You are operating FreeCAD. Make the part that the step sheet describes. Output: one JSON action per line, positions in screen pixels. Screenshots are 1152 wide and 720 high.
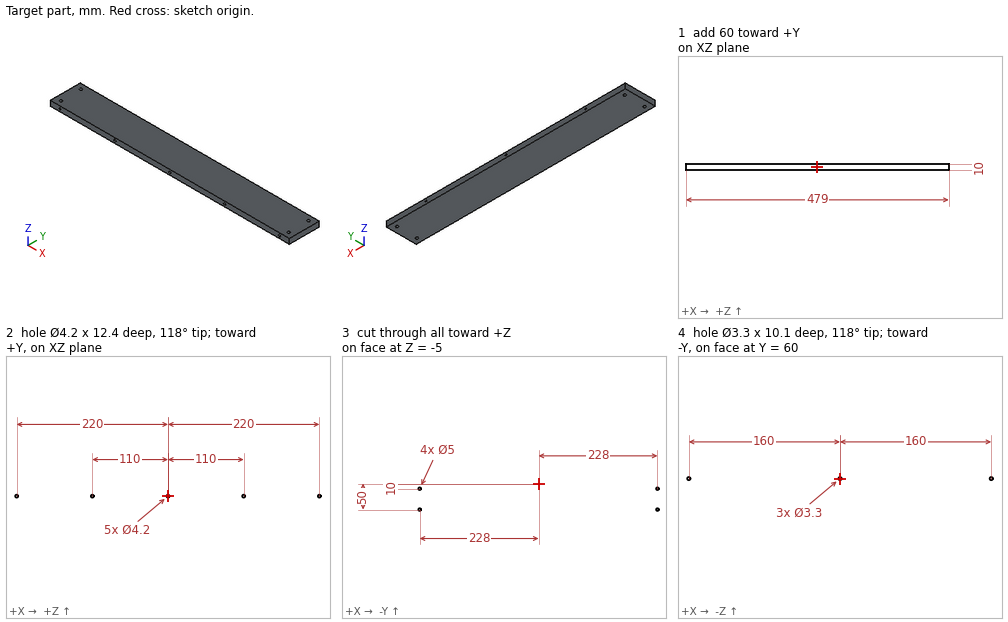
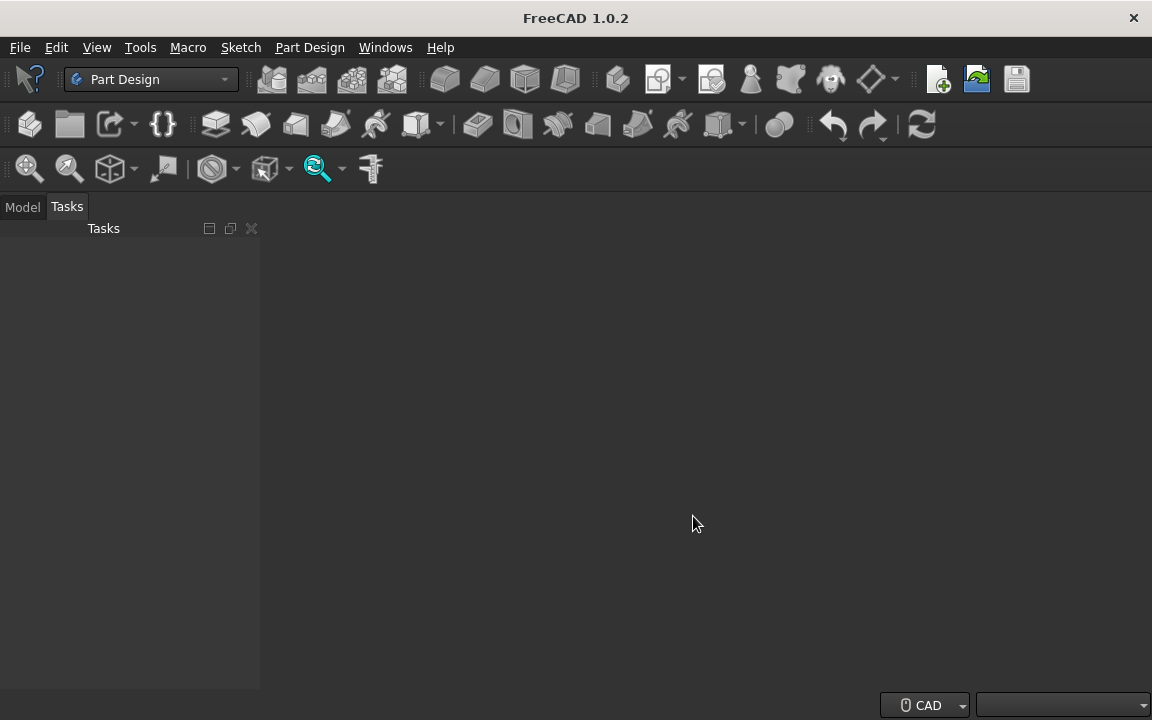
{"action": "left_click", "coordinate": [938, 80]}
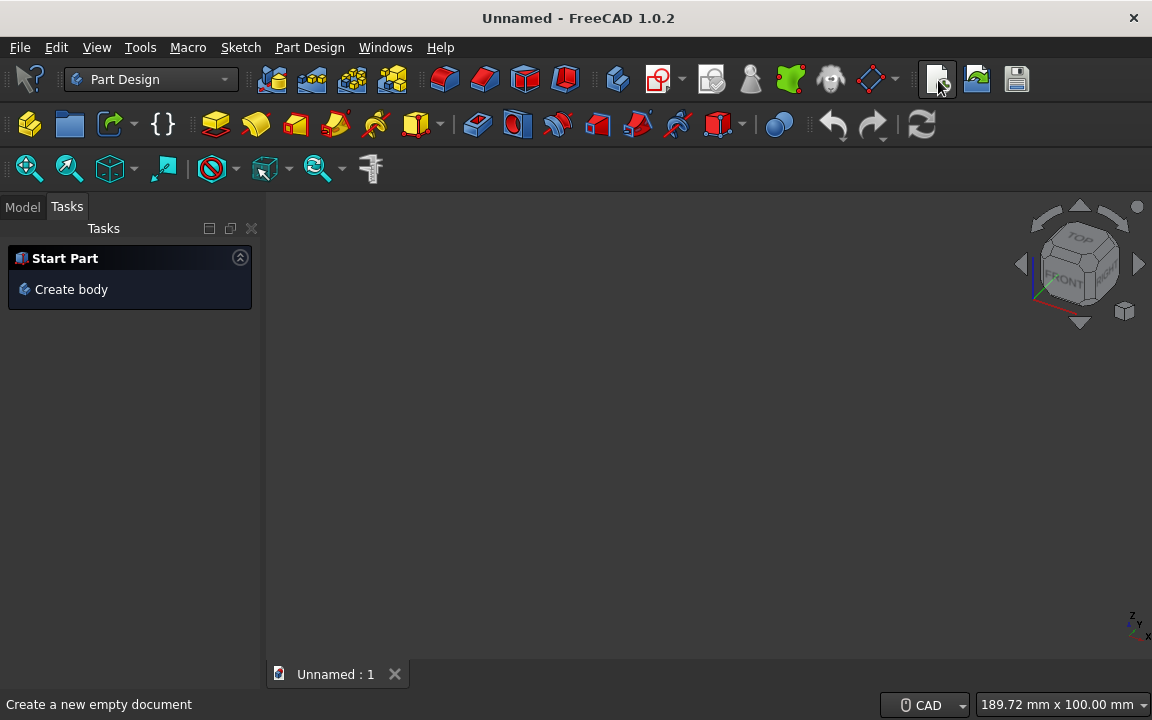
{"action": "left_click", "coordinate": [658, 80]}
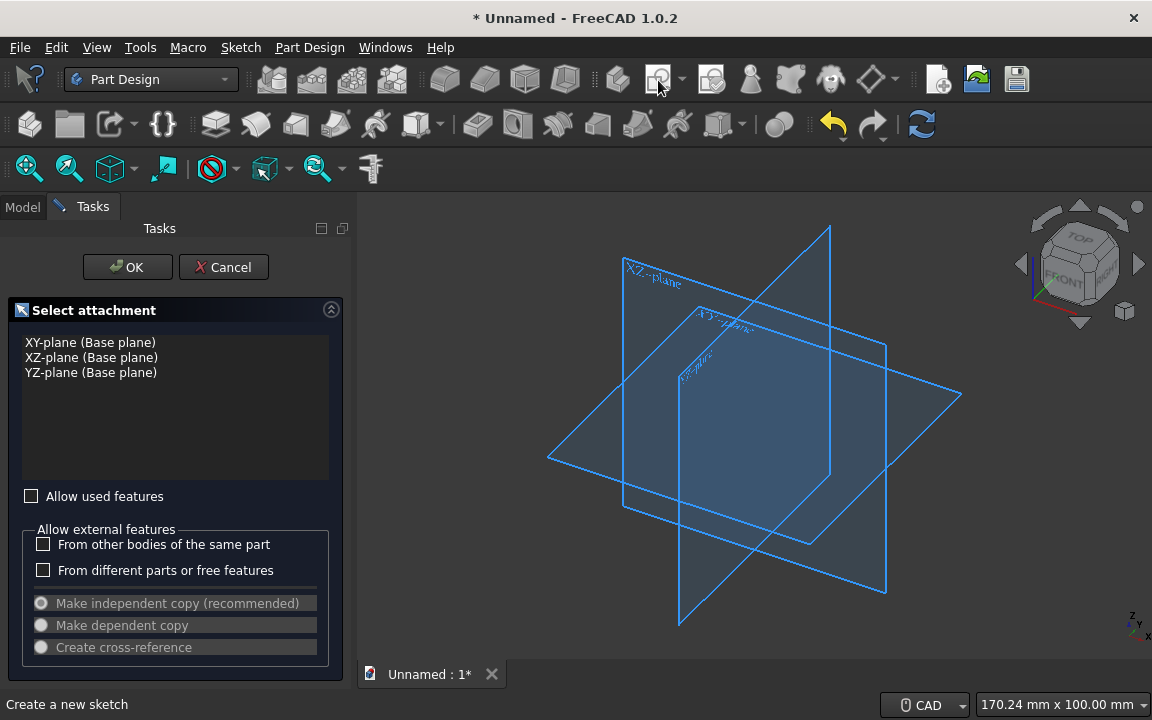
{"action": "left_click", "coordinate": [82, 358]}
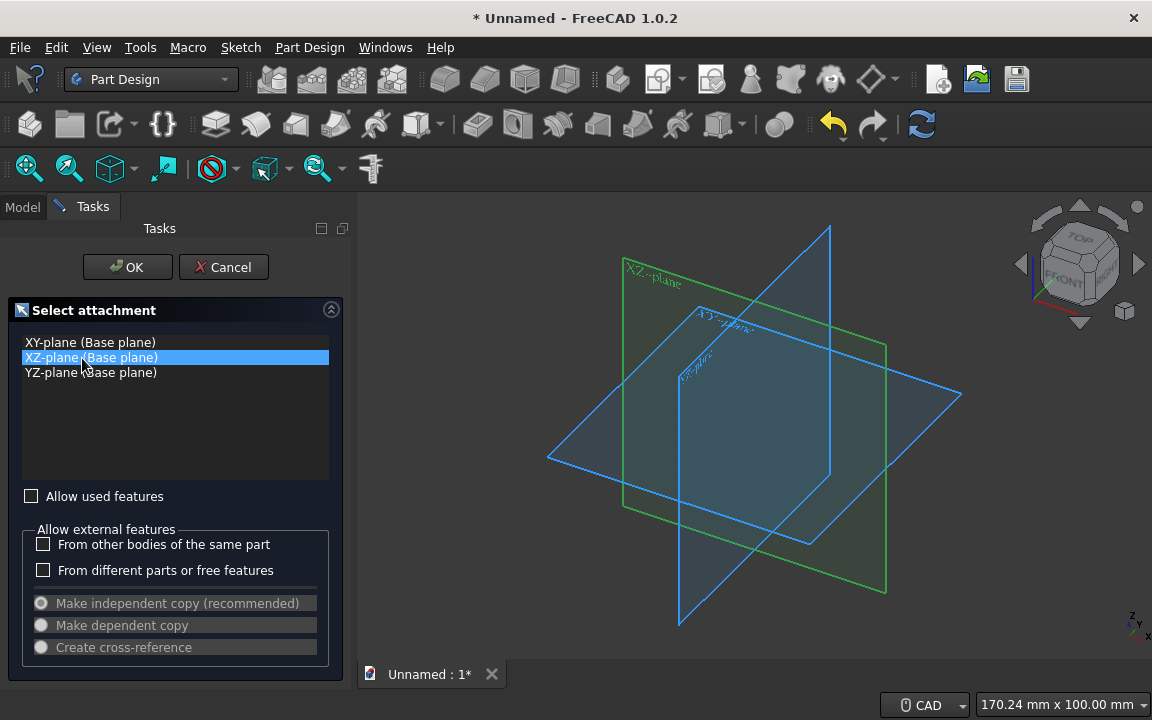
{"action": "left_click", "coordinate": [128, 267]}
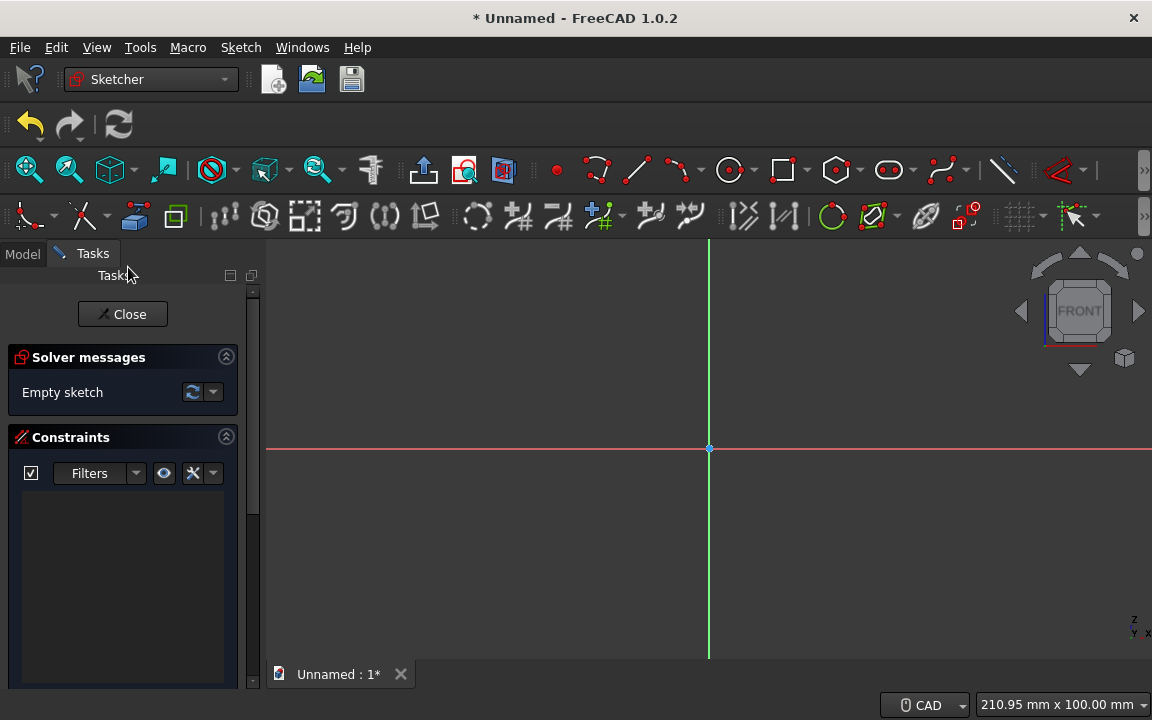
{"action": "scroll", "coordinate": [618, 449], "scroll_direction": "down", "scroll_amount": 7}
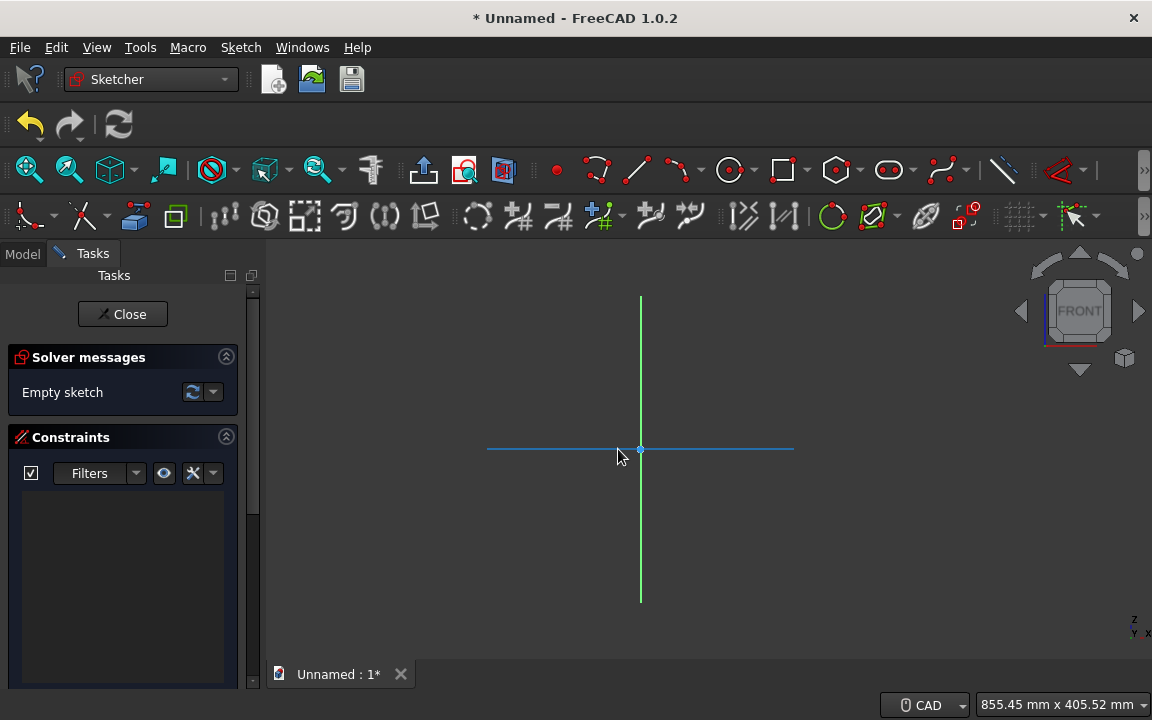
{"action": "left_click", "coordinate": [810, 170]}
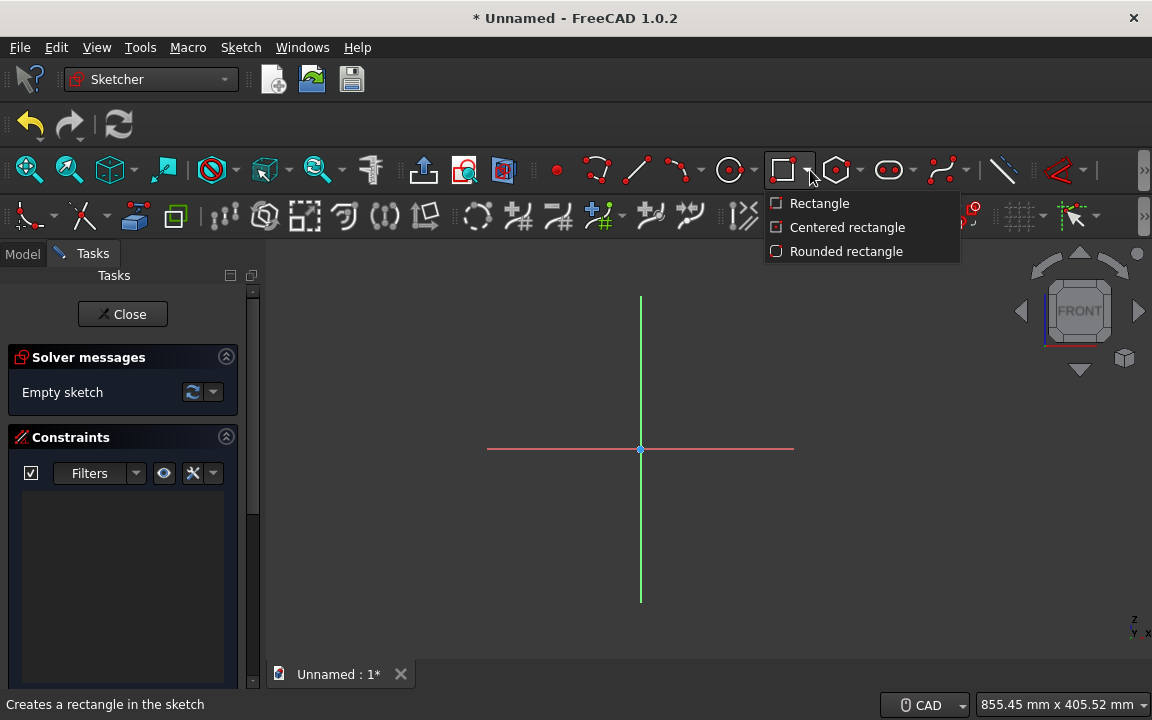
{"action": "left_click", "coordinate": [862, 227]}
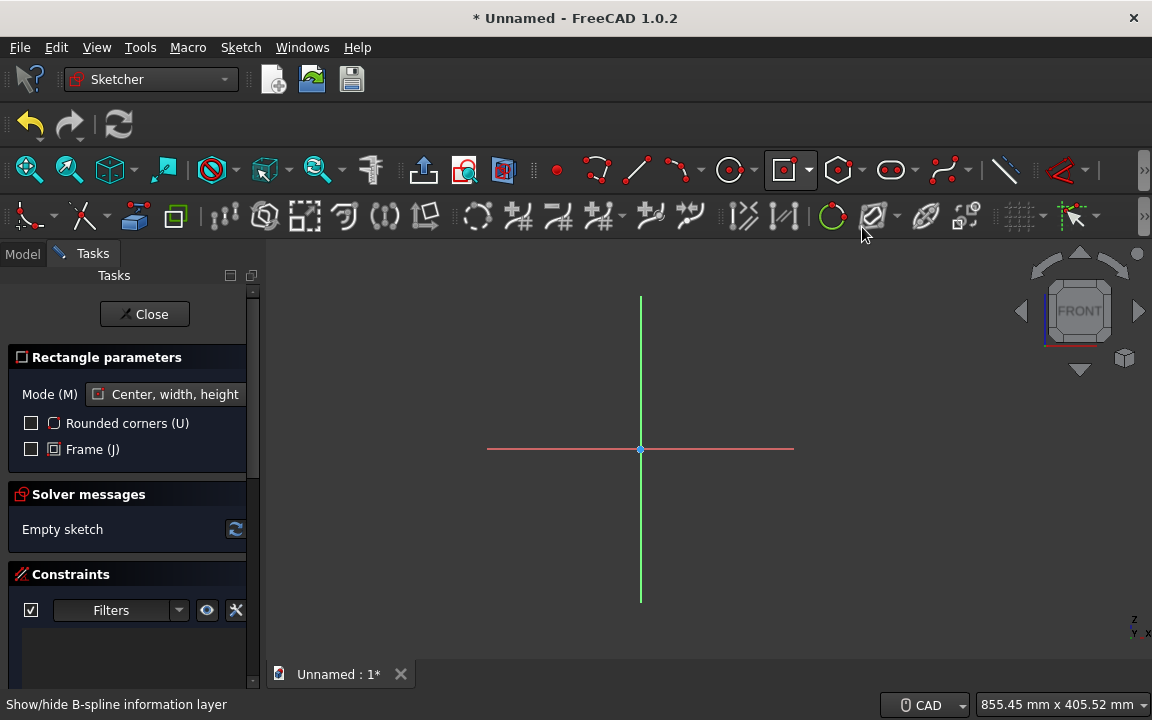
{"action": "scroll", "coordinate": [641, 449], "scroll_direction": "up", "scroll_amount": 6}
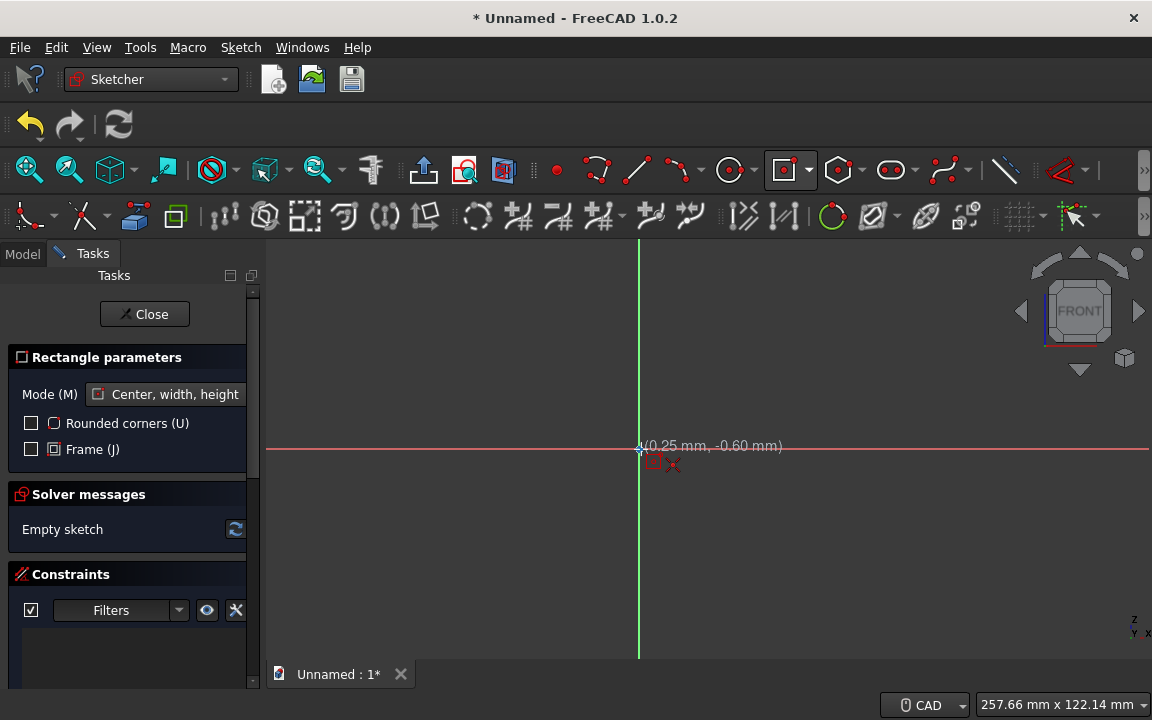
{"action": "left_click", "coordinate": [639, 449]}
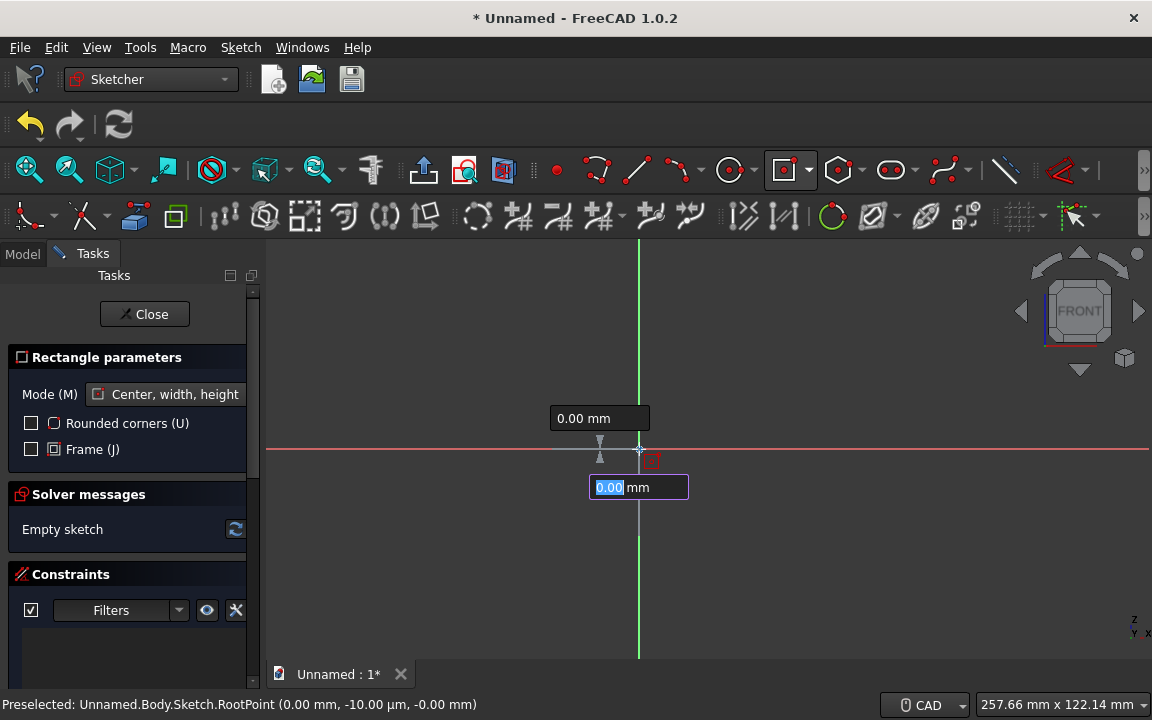
{"action": "scroll", "coordinate": [641, 449], "scroll_direction": "down", "scroll_amount": 6}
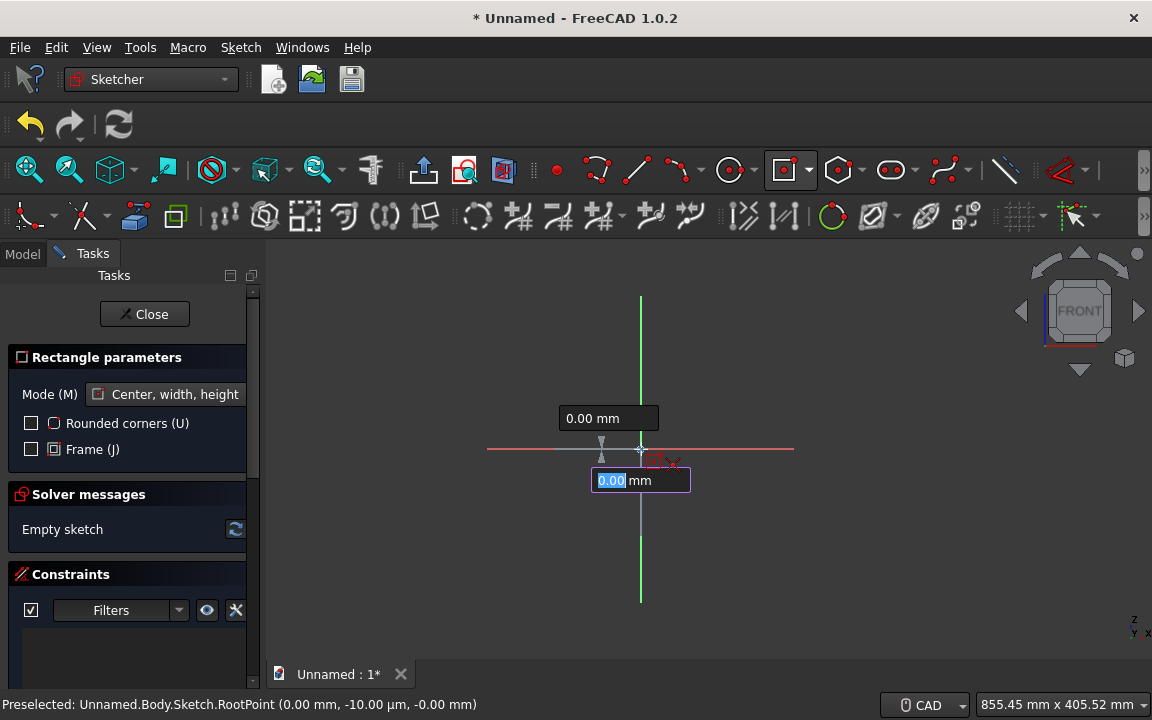
{"action": "scroll", "coordinate": [889, 444], "scroll_direction": "up", "scroll_amount": 6}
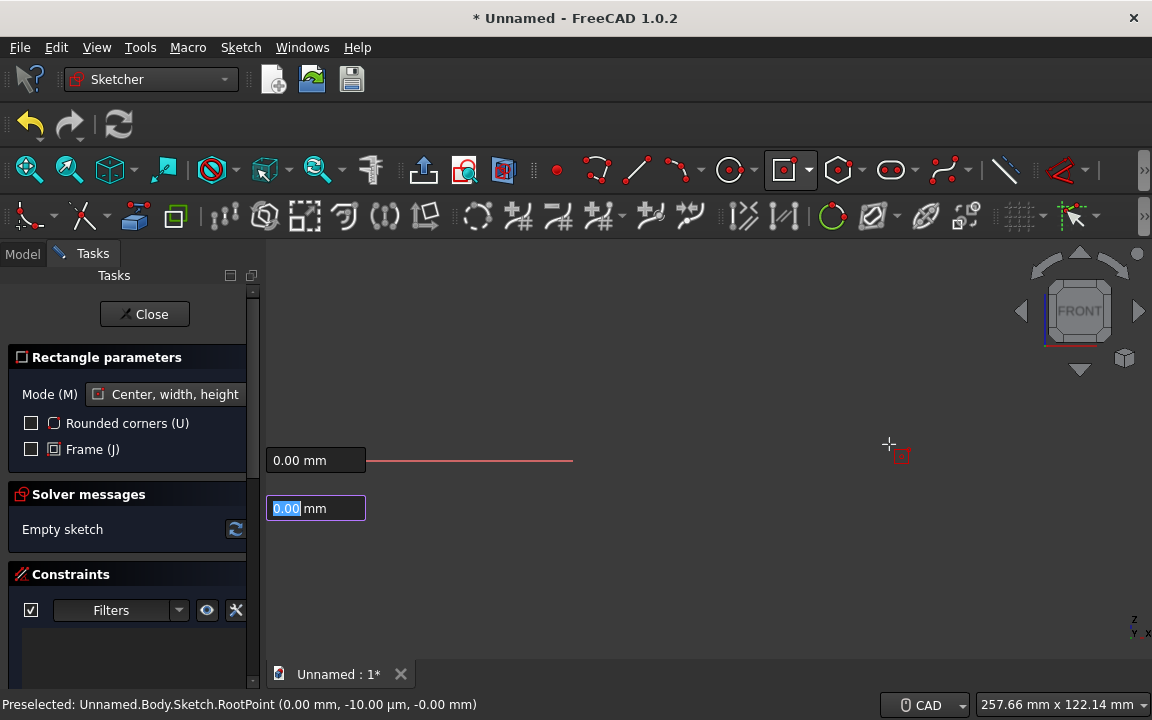
{"action": "left_click", "coordinate": [887, 444]}
{"action": "key", "text": "Escape"}